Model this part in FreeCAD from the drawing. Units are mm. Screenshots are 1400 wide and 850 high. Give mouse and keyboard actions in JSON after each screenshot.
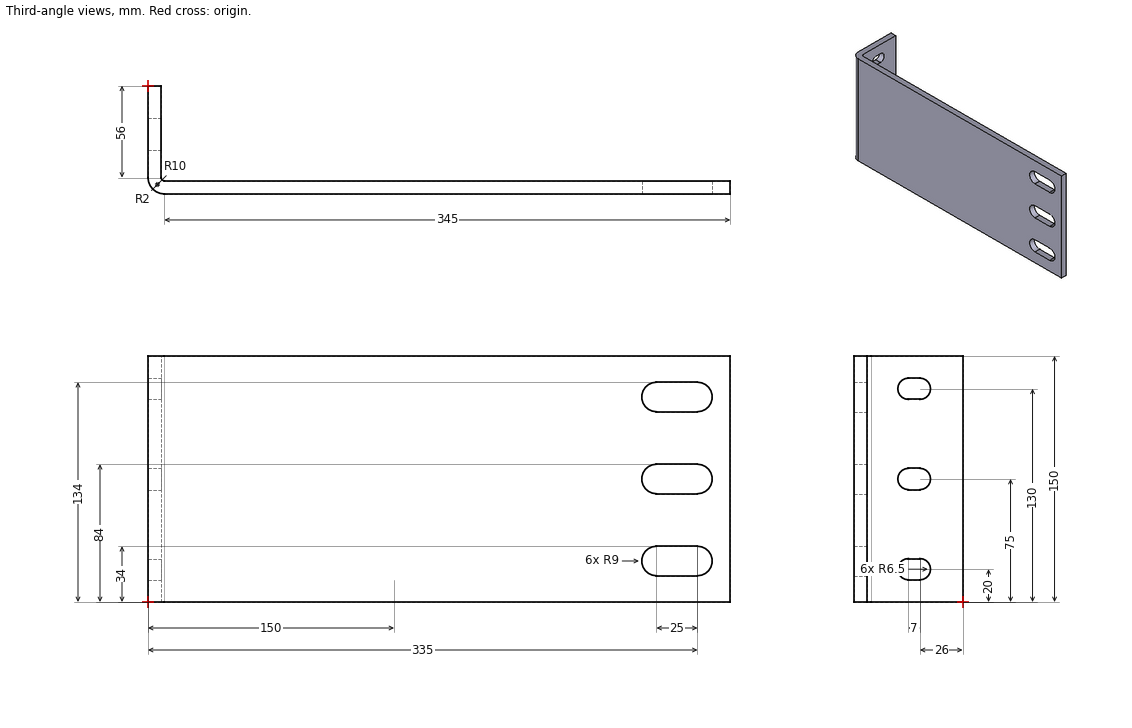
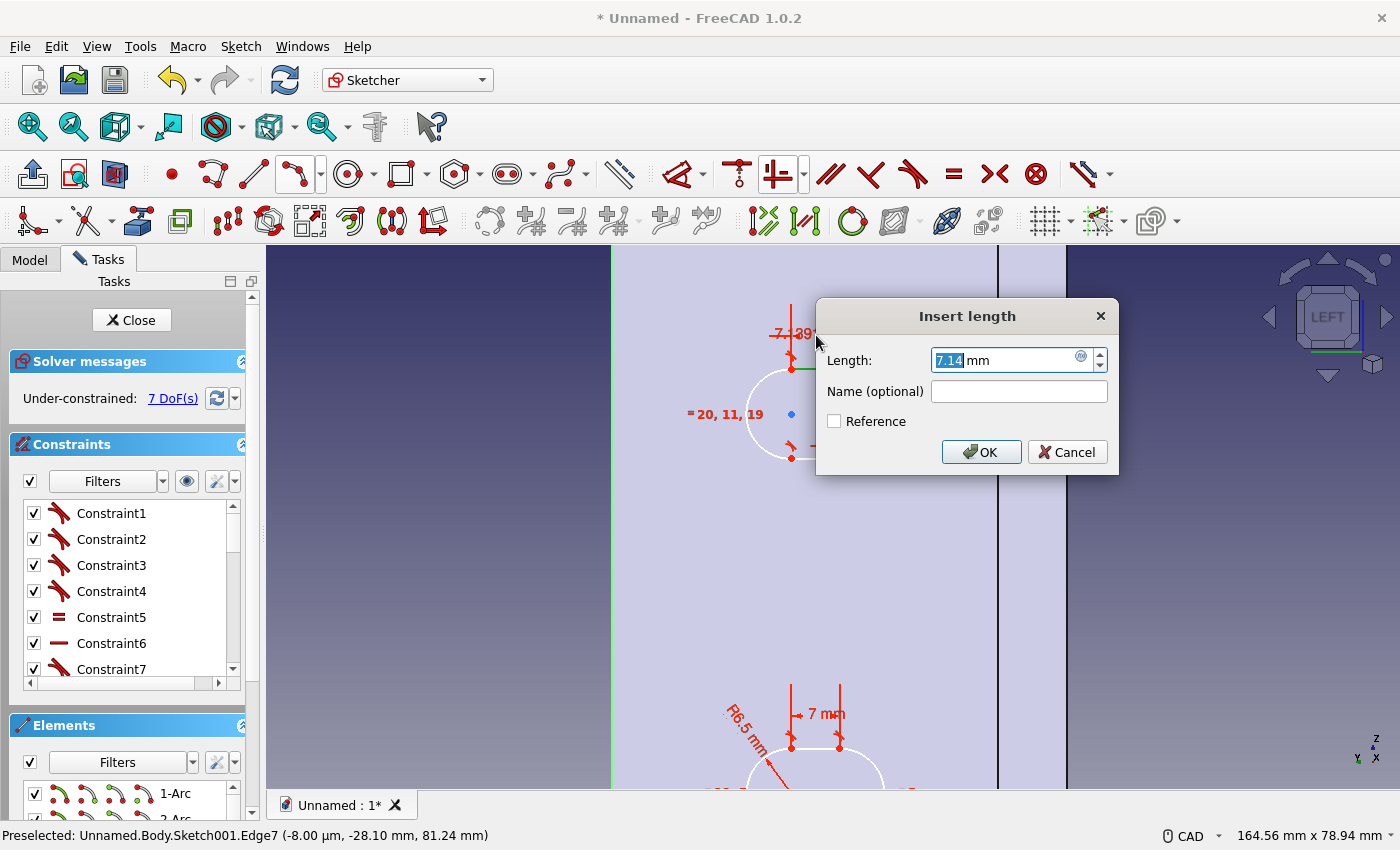
{"action": "type", "text": "7"}
{"action": "key", "text": "Return"}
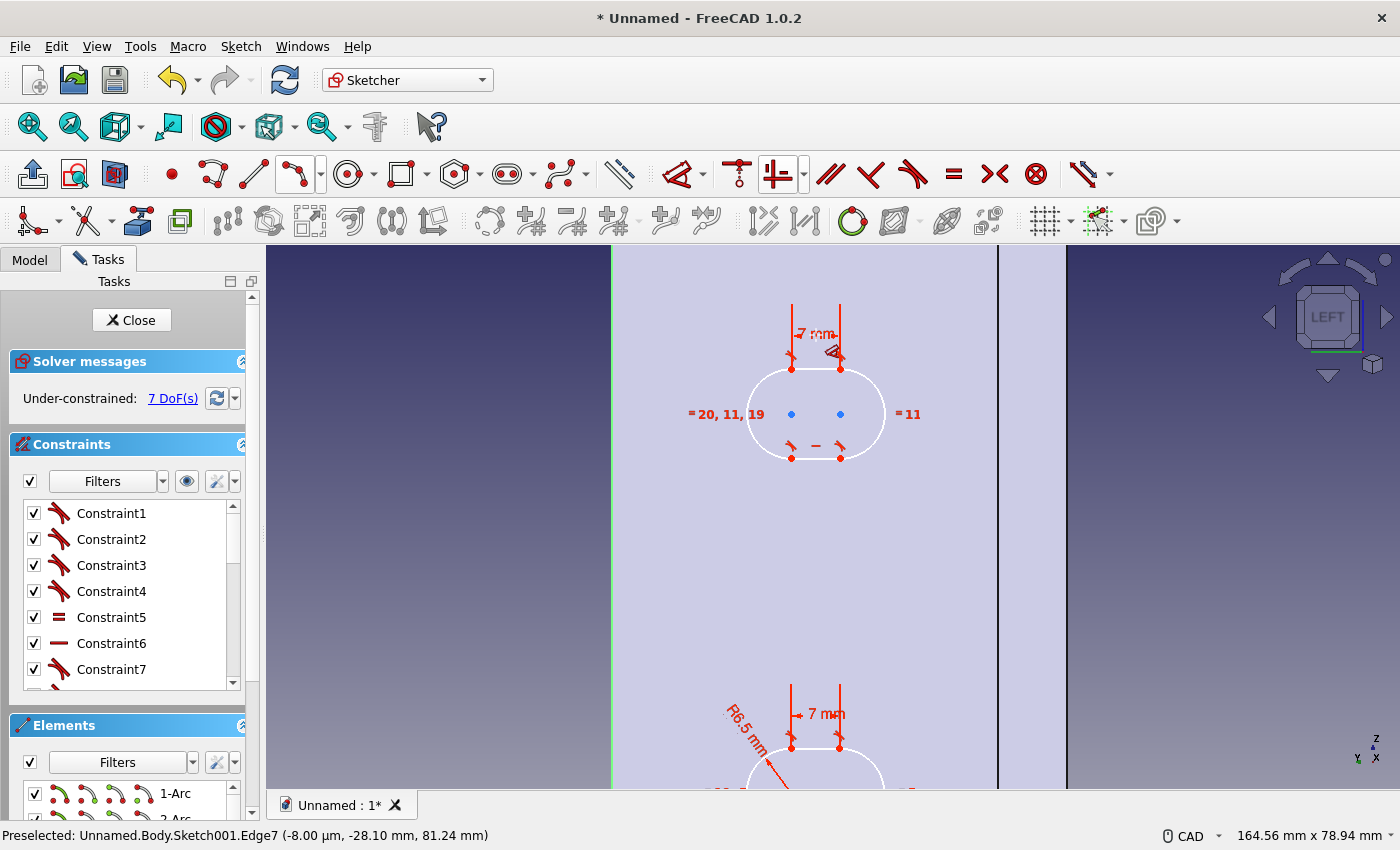
{"action": "scroll", "coordinate": [774, 551], "scroll_direction": "down", "scroll_amount": 5}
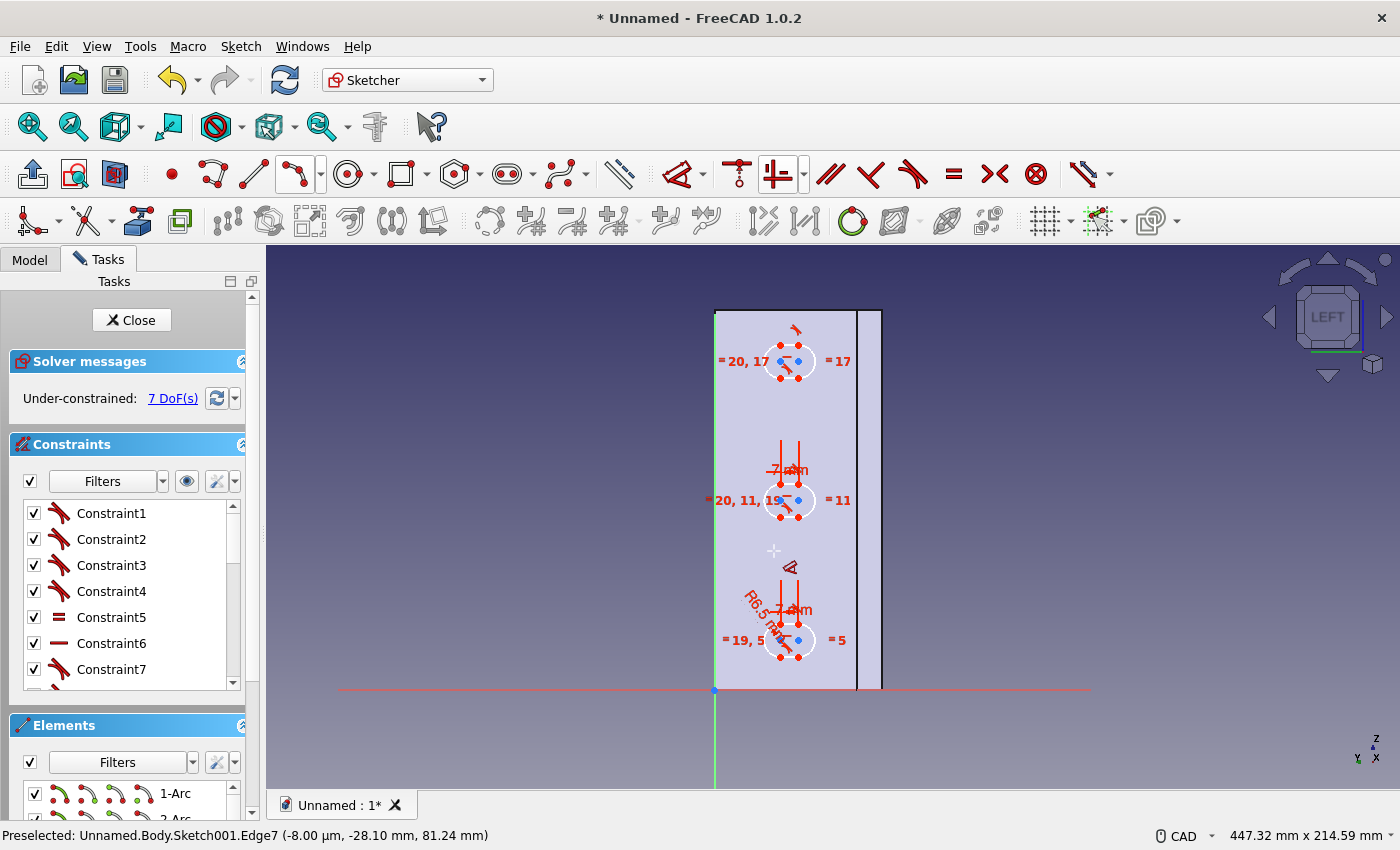
{"action": "scroll", "coordinate": [786, 345], "scroll_direction": "up", "scroll_amount": 5}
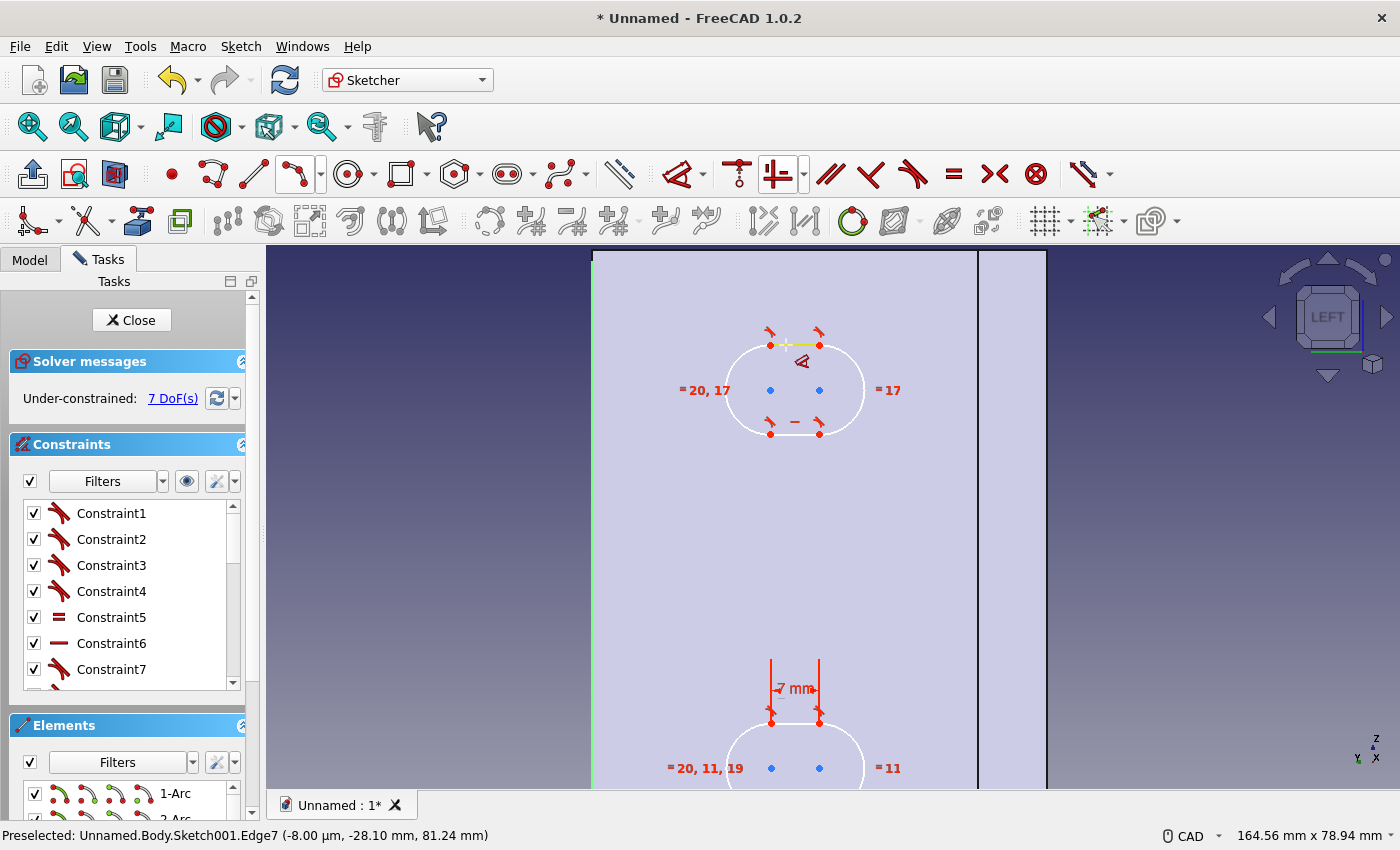
{"action": "left_click", "coordinate": [785, 345]}
{"action": "left_click", "coordinate": [795, 311]}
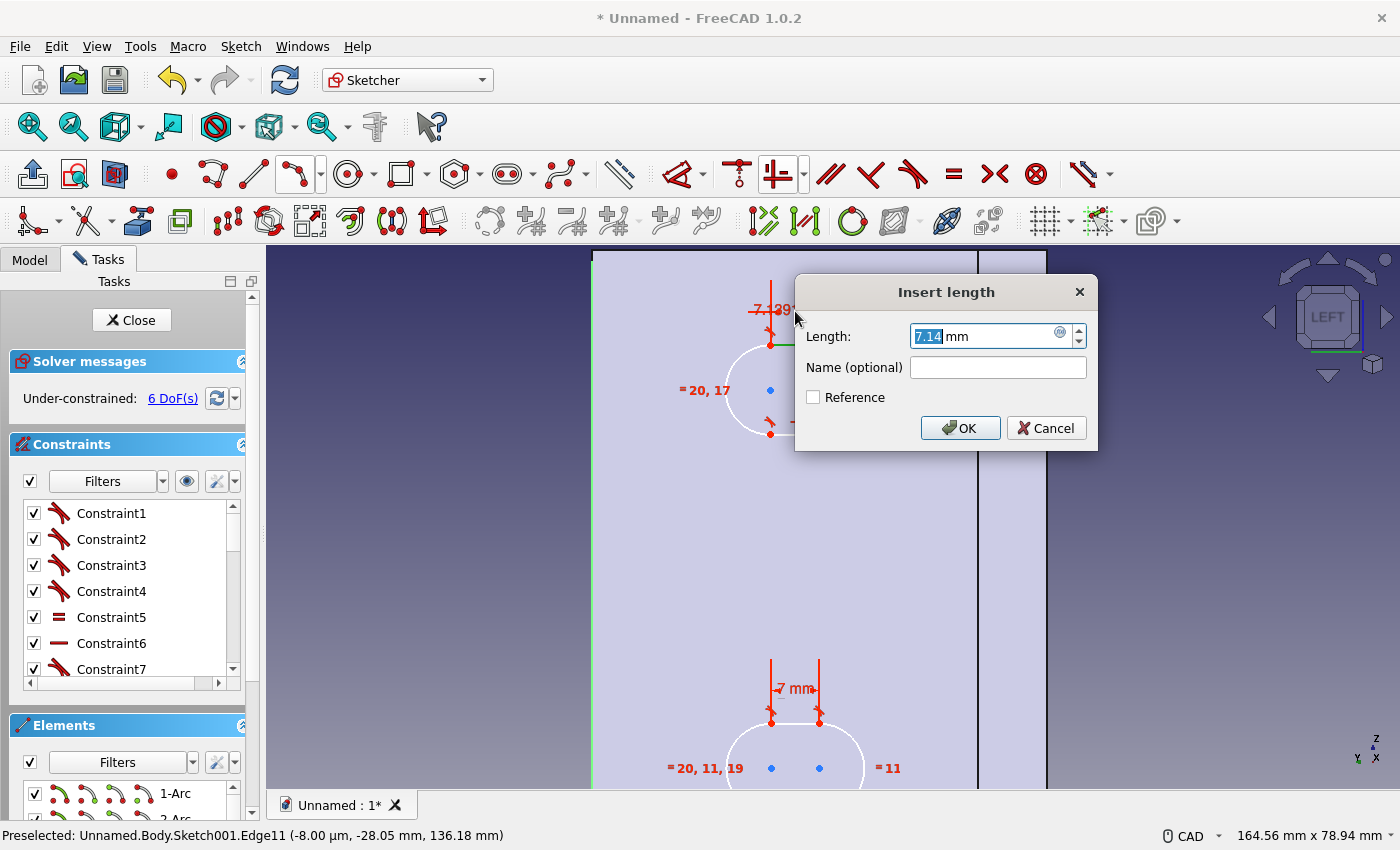
{"action": "type", "text": "7"}
{"action": "key", "text": "Return"}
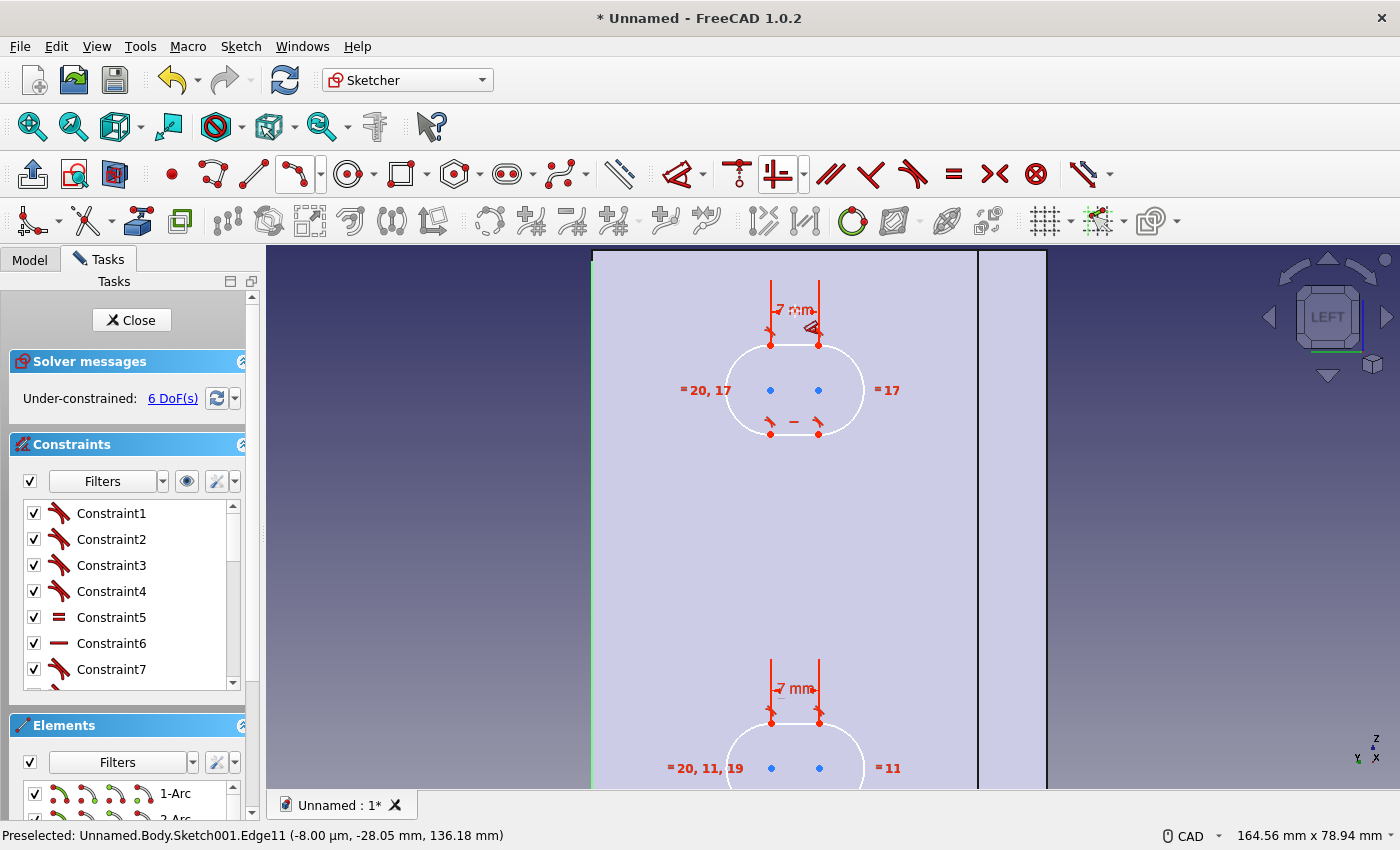
{"action": "scroll", "coordinate": [786, 345], "scroll_direction": "down", "scroll_amount": 5}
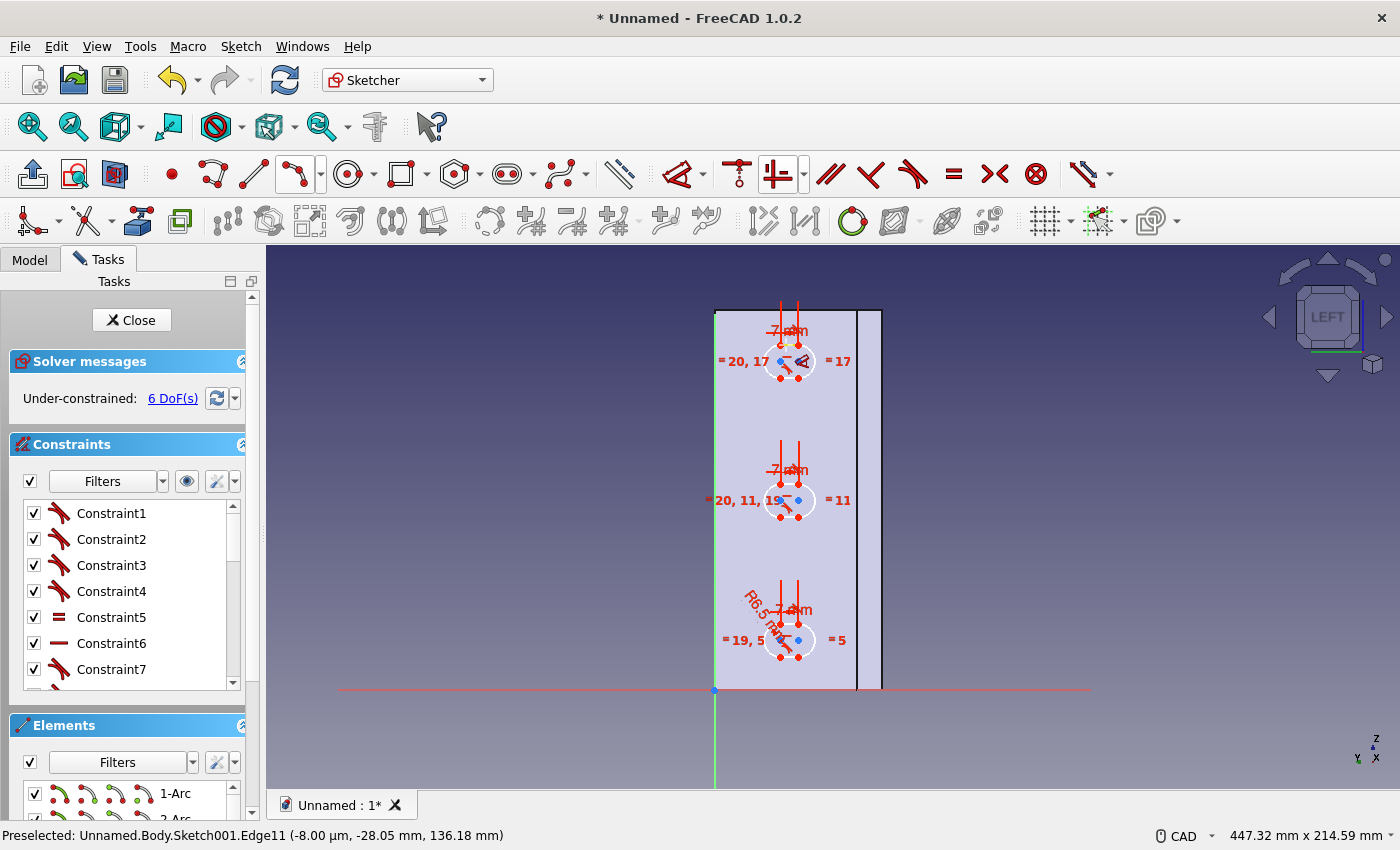
{"action": "left_click", "coordinate": [781, 624]}
{"action": "left_click", "coordinate": [748, 724]}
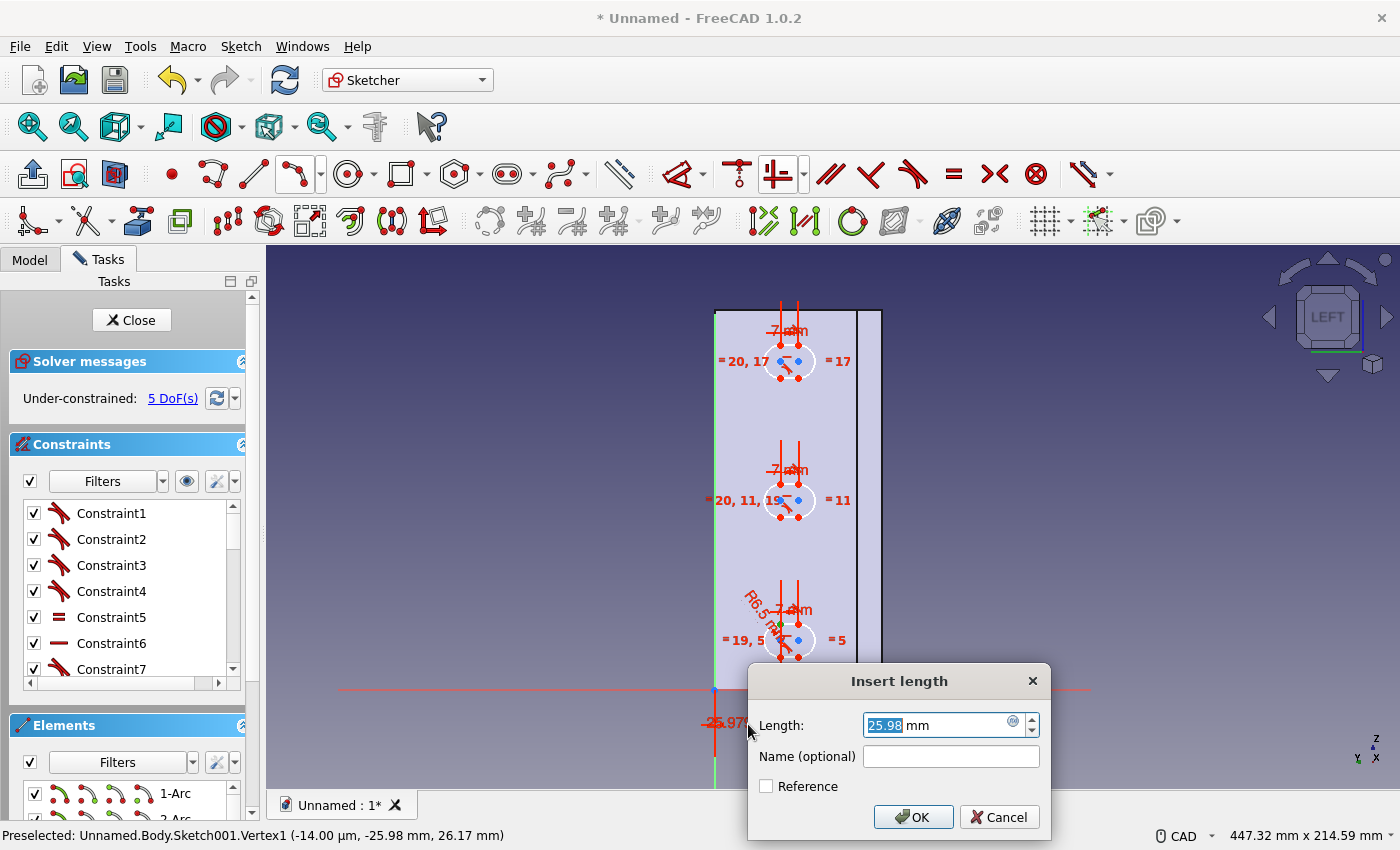
{"action": "type", "text": "26"}
{"action": "key", "text": "Return"}